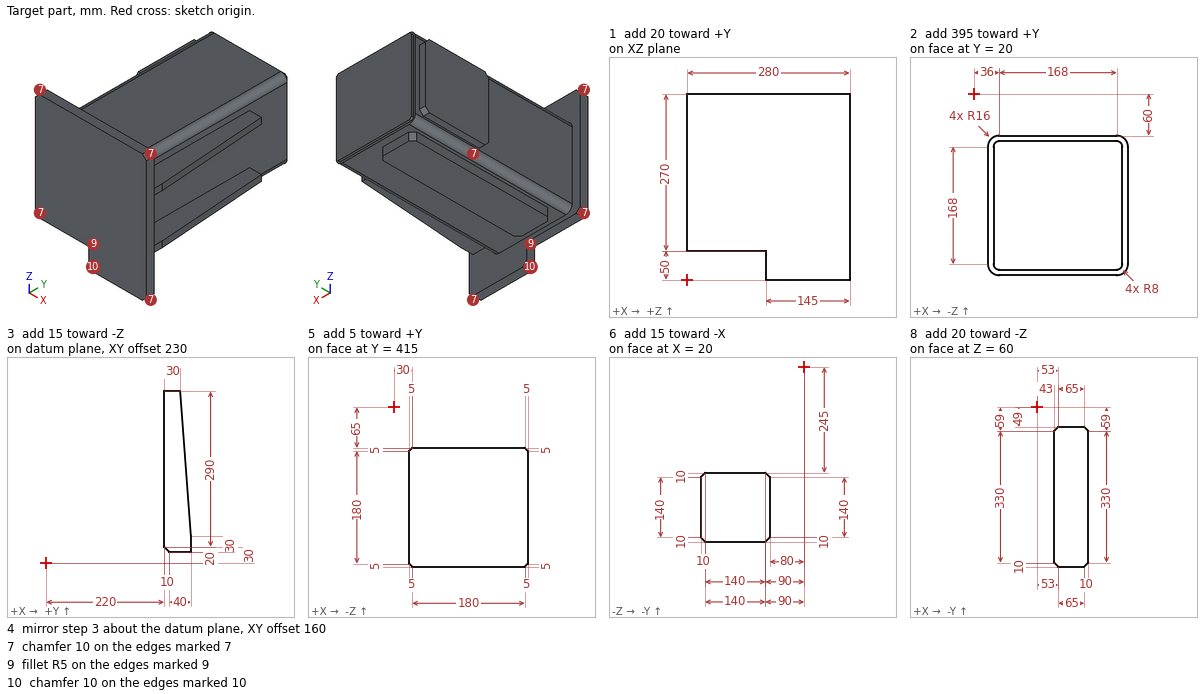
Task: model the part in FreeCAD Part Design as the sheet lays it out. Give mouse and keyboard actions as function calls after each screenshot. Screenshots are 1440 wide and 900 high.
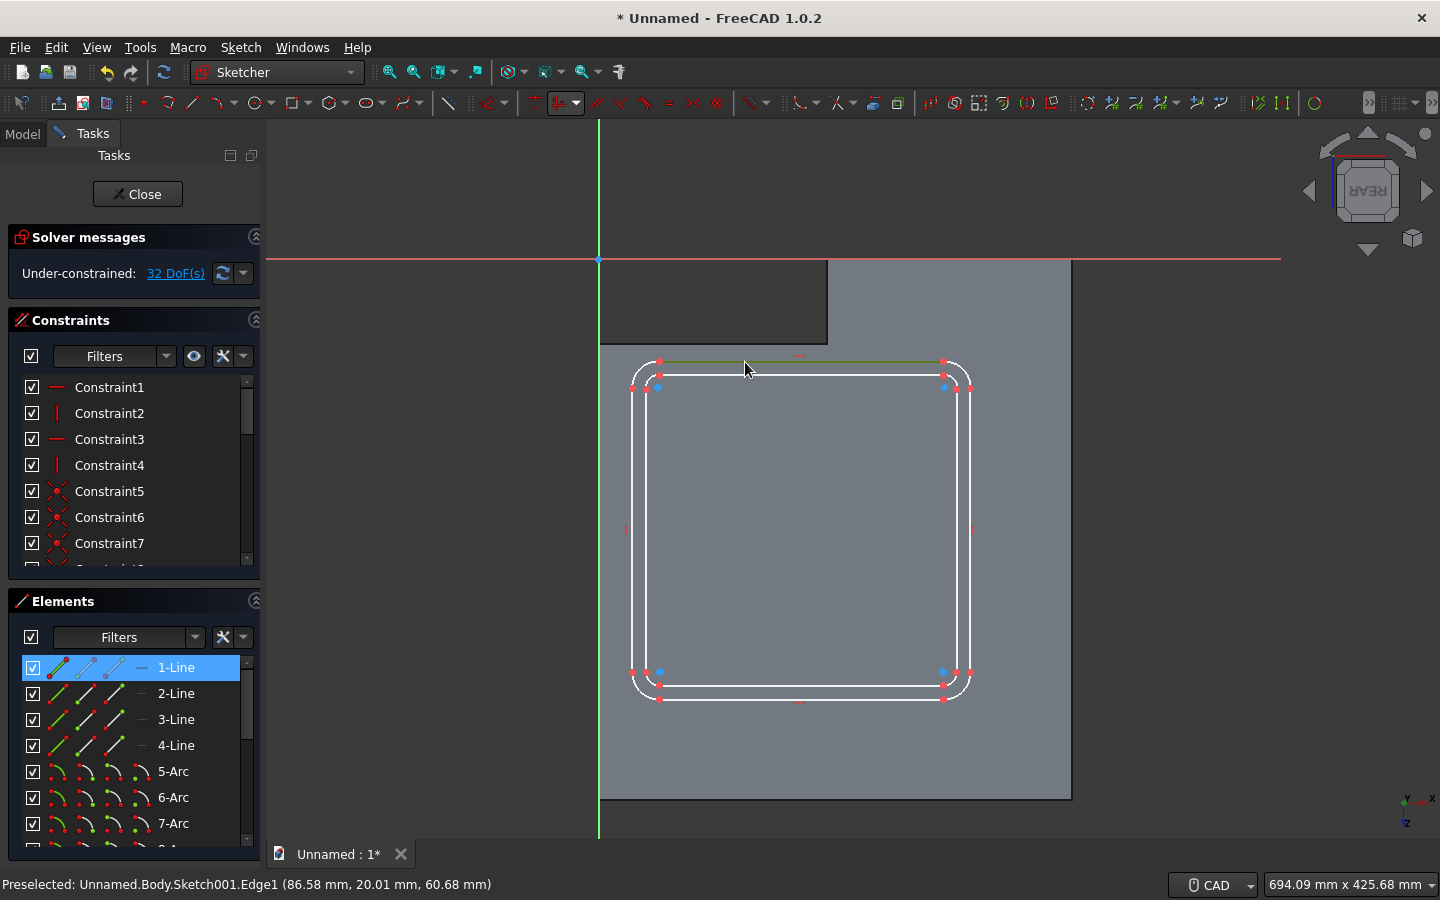
click(647, 364)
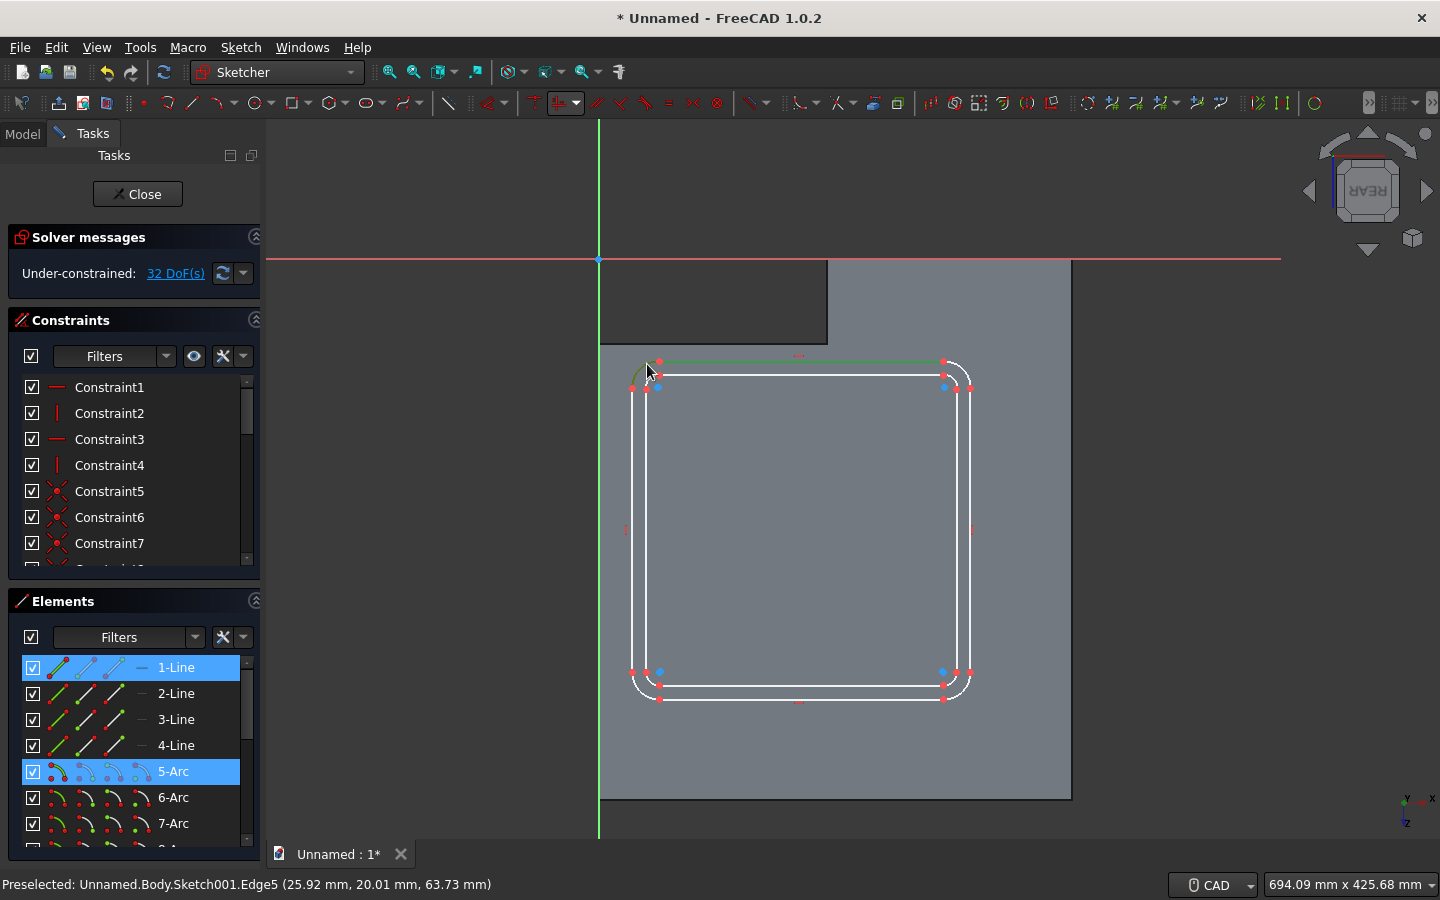
click(646, 104)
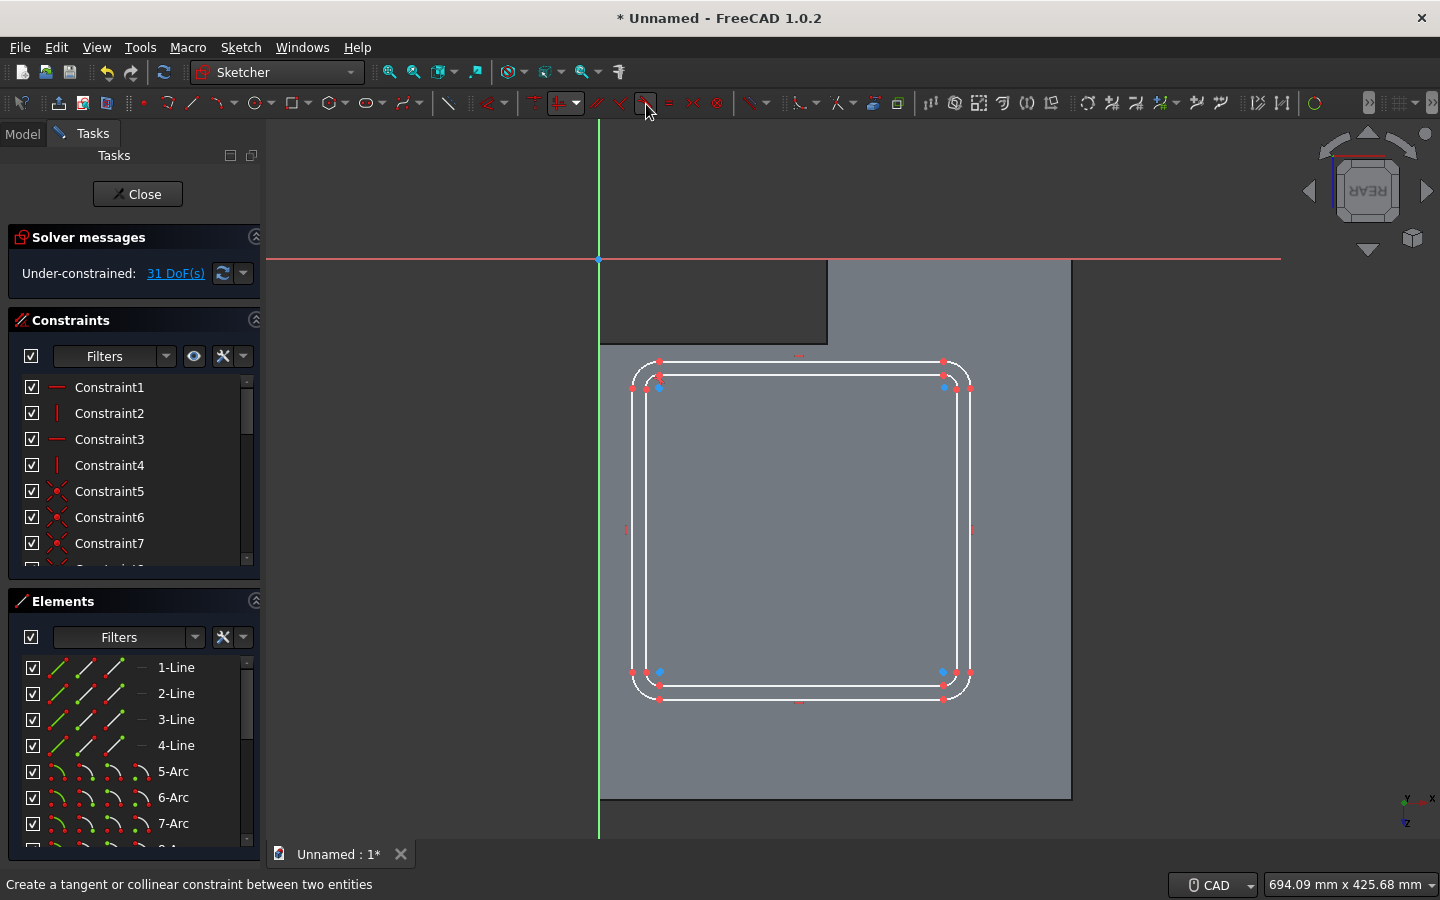
click(858, 362)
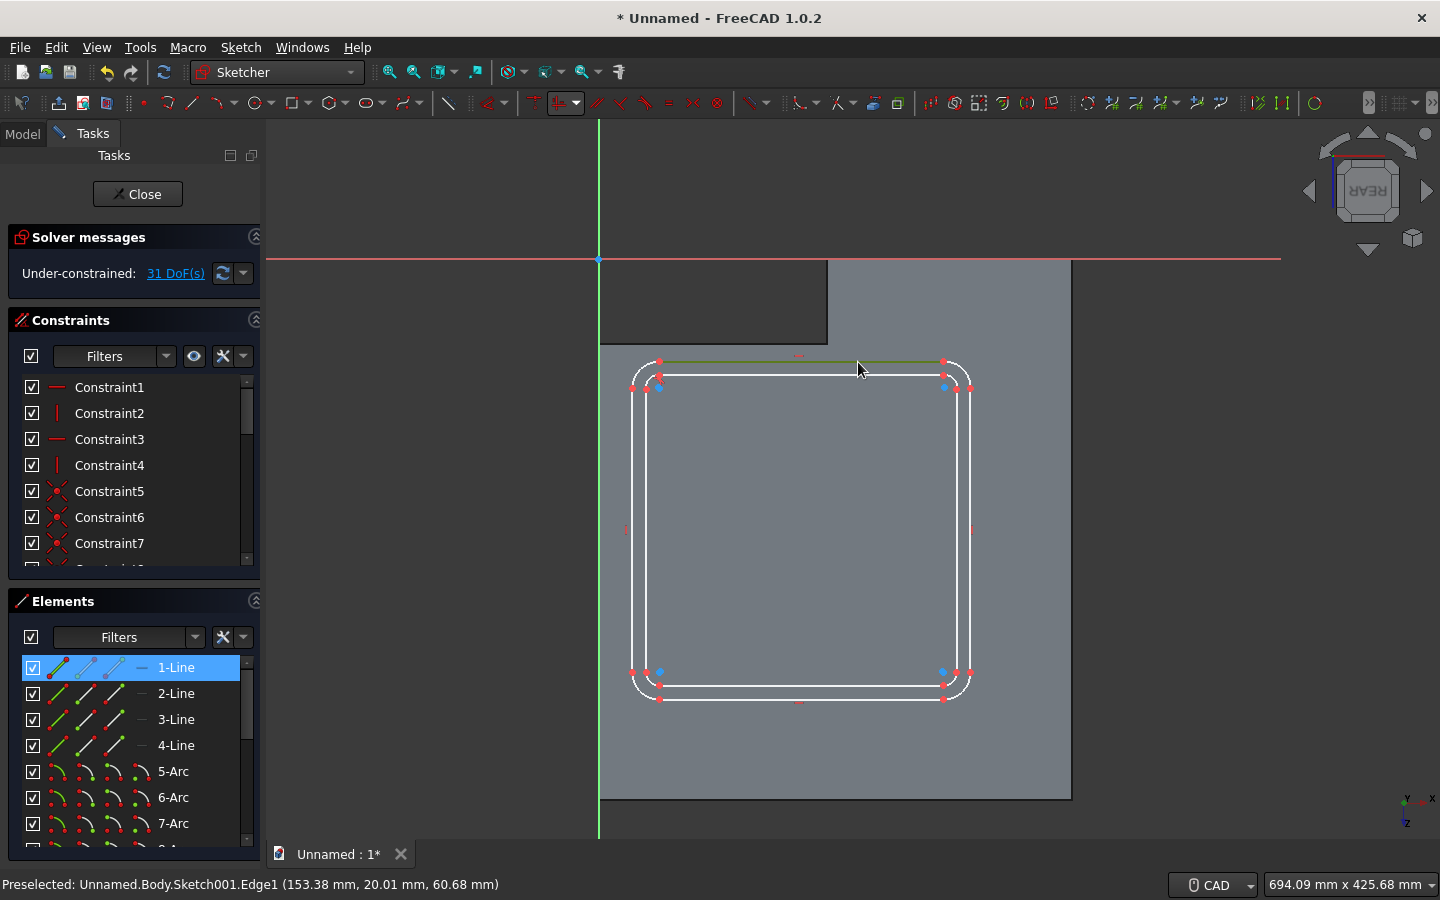
click(968, 376)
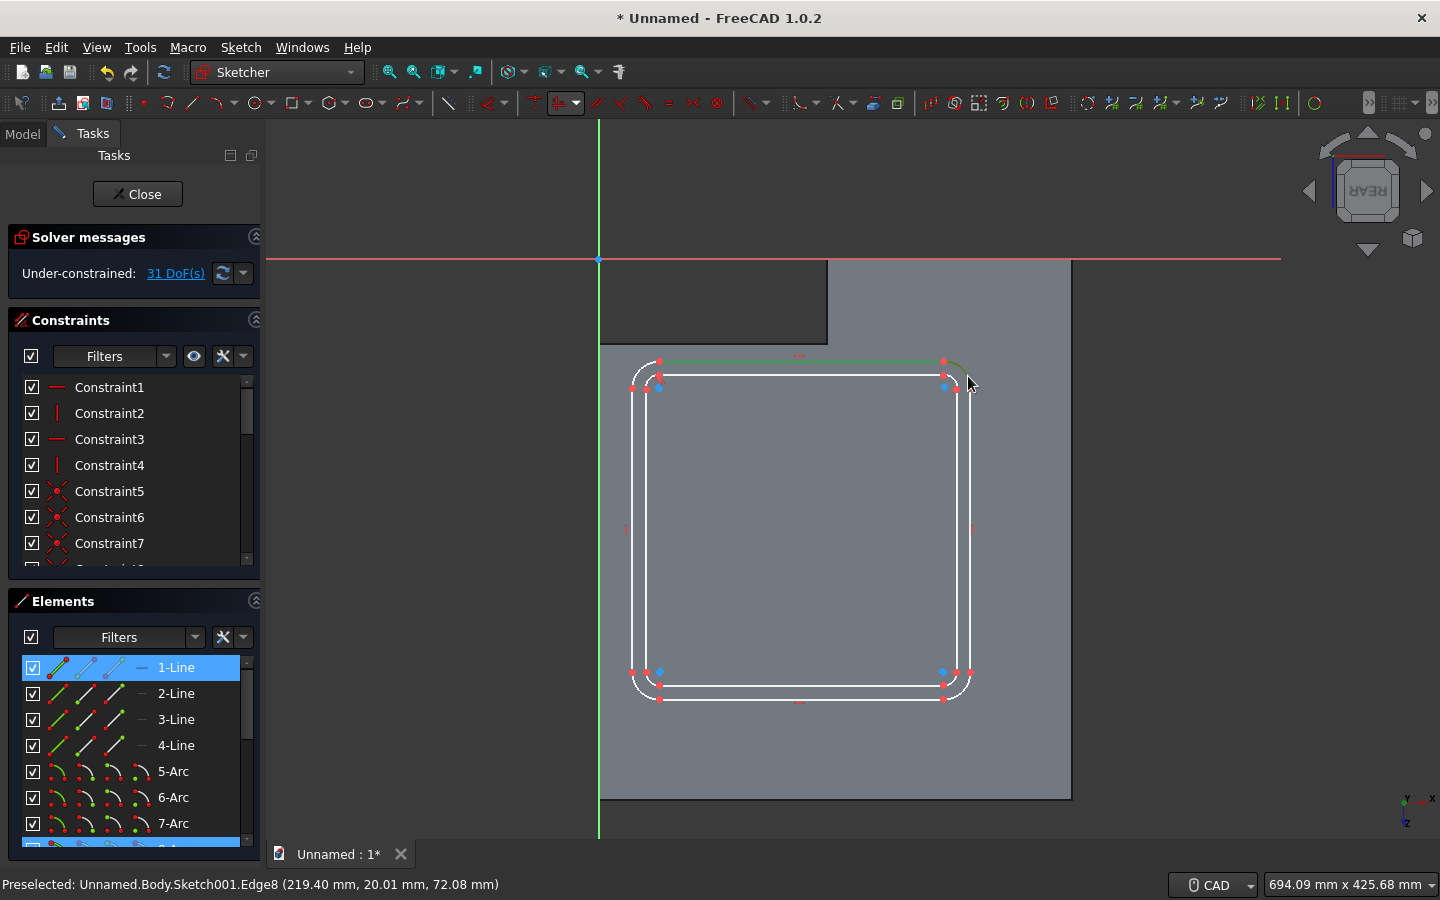
click(646, 104)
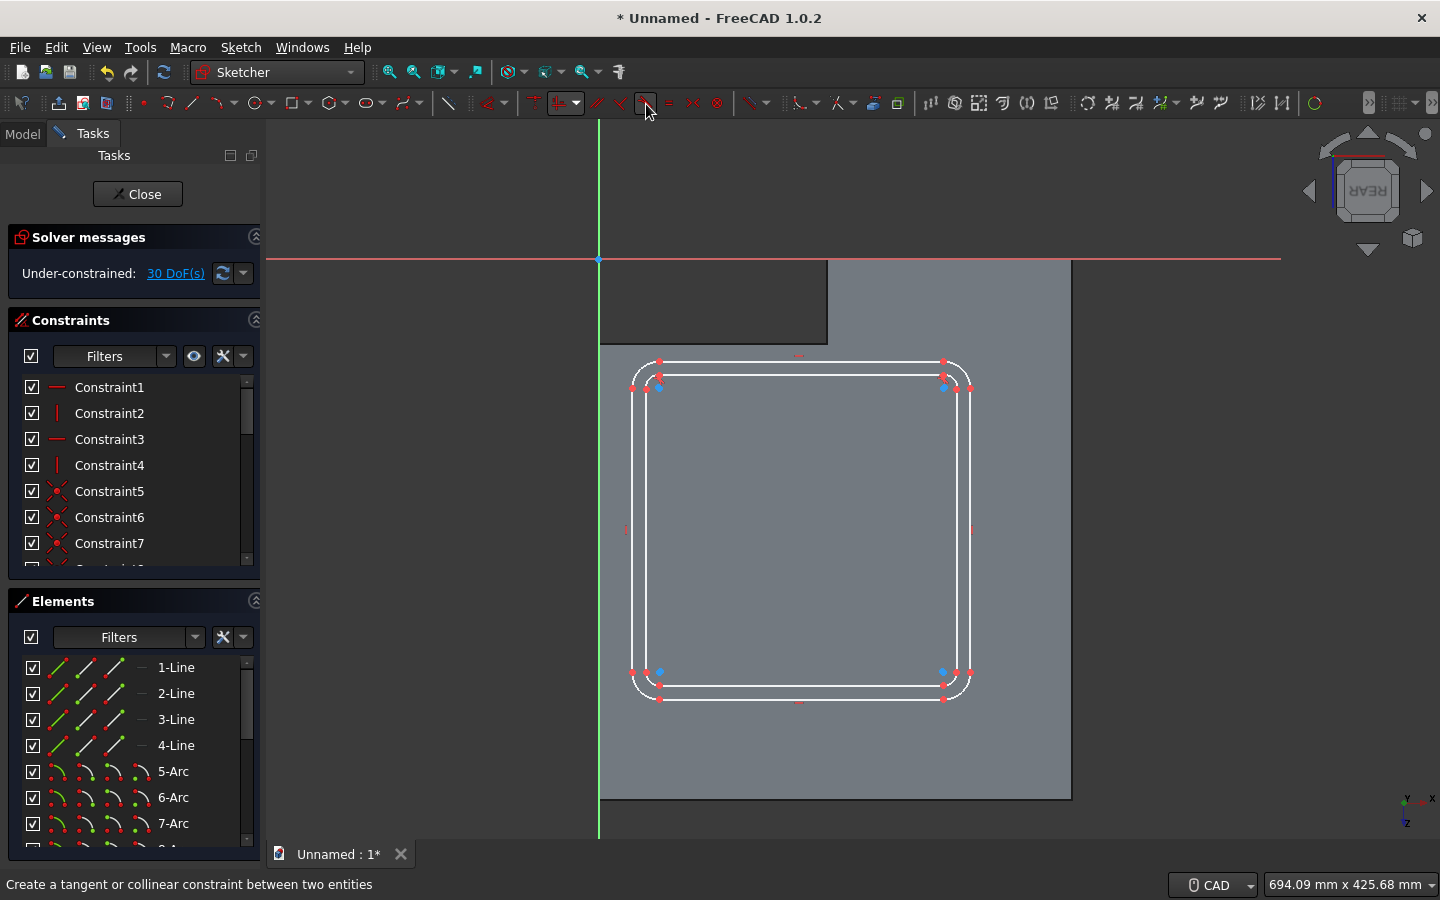
click(632, 474)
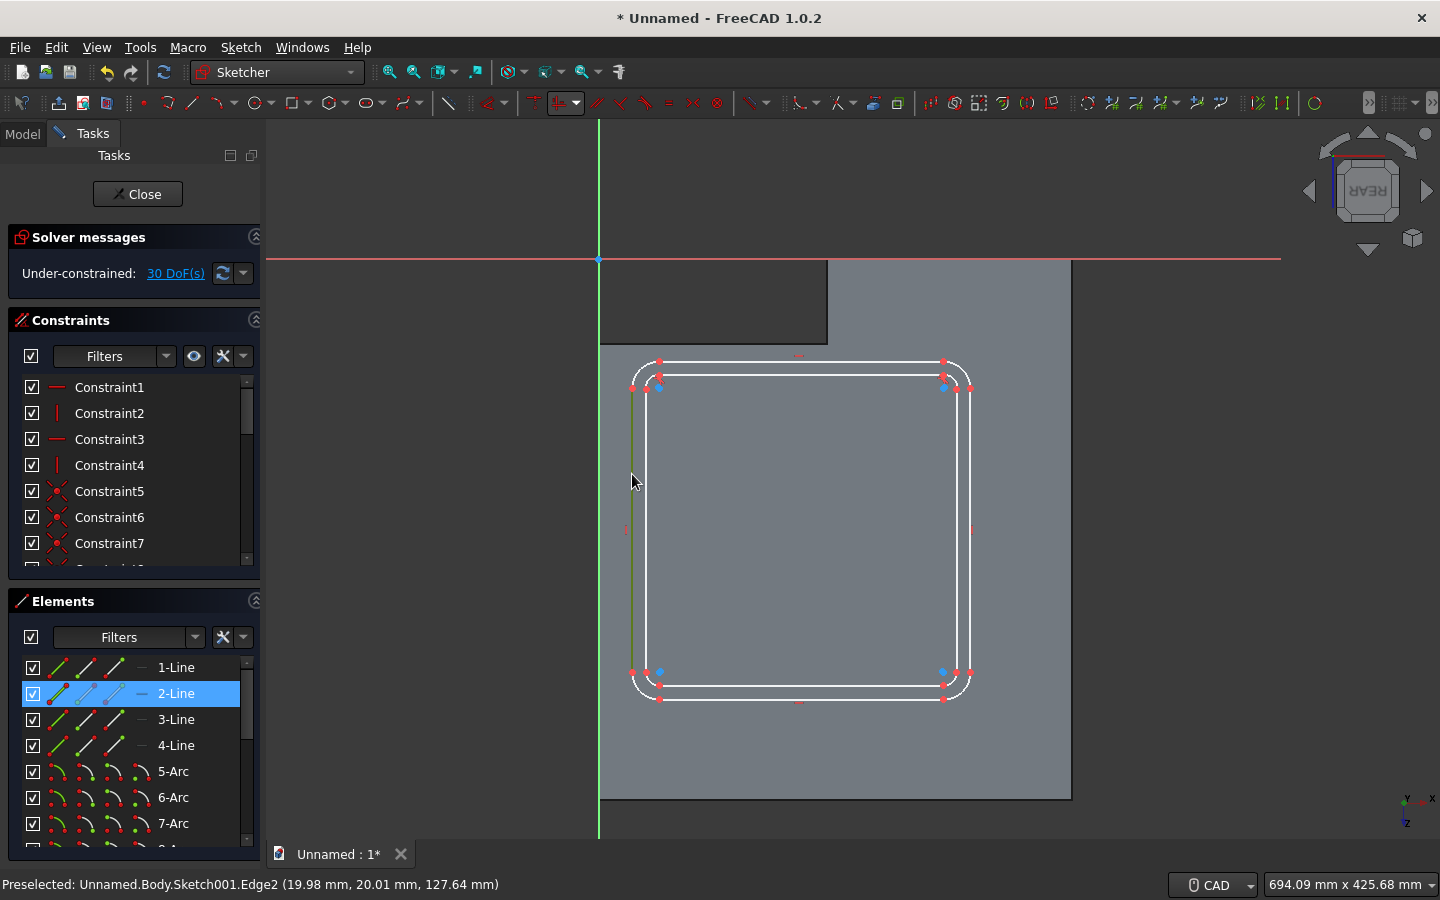
click(647, 365)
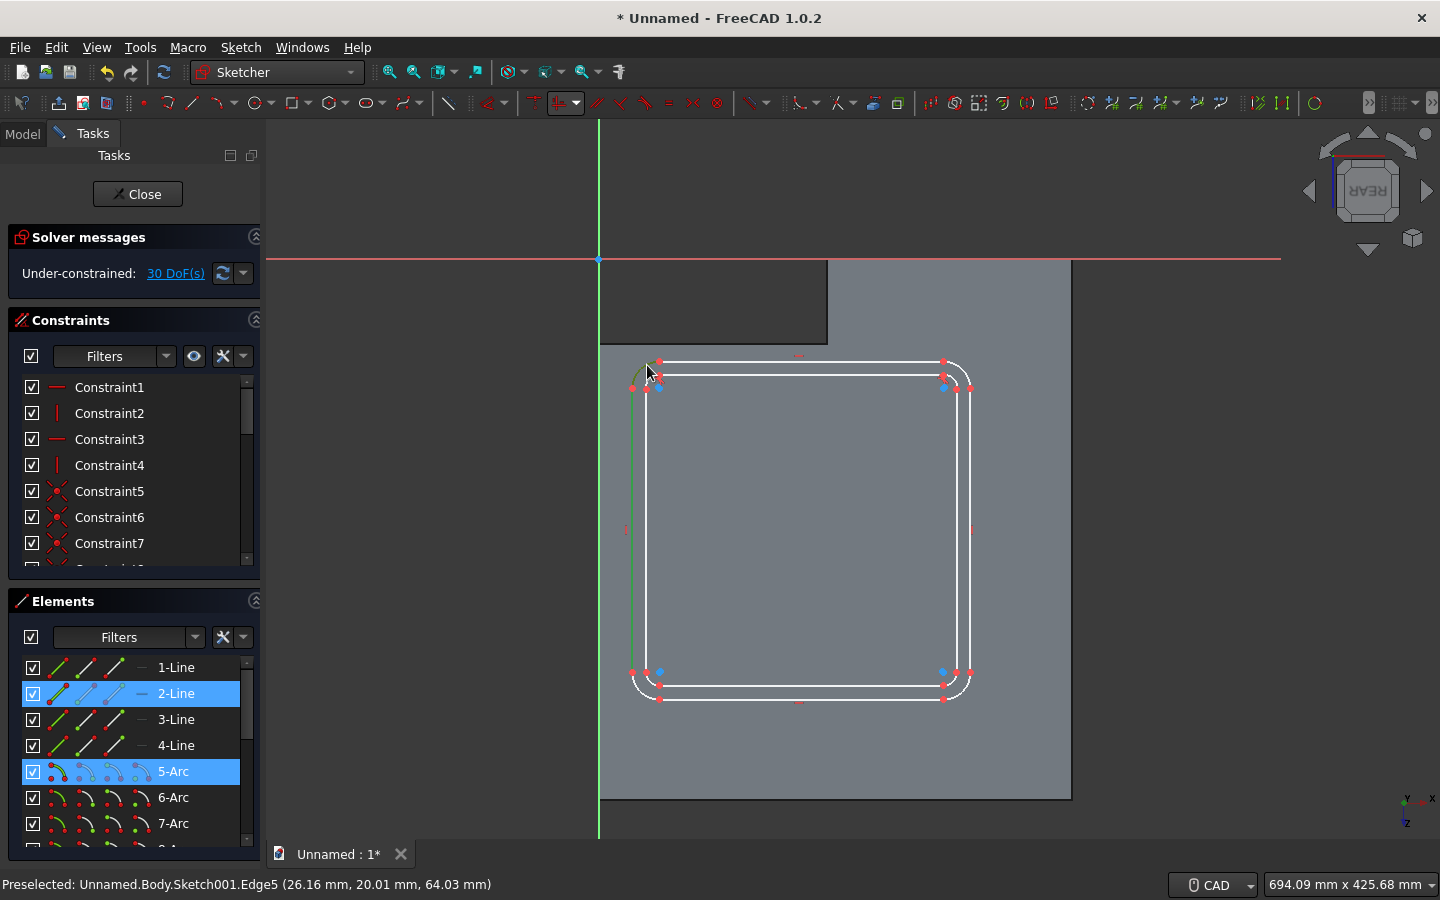
click(646, 104)